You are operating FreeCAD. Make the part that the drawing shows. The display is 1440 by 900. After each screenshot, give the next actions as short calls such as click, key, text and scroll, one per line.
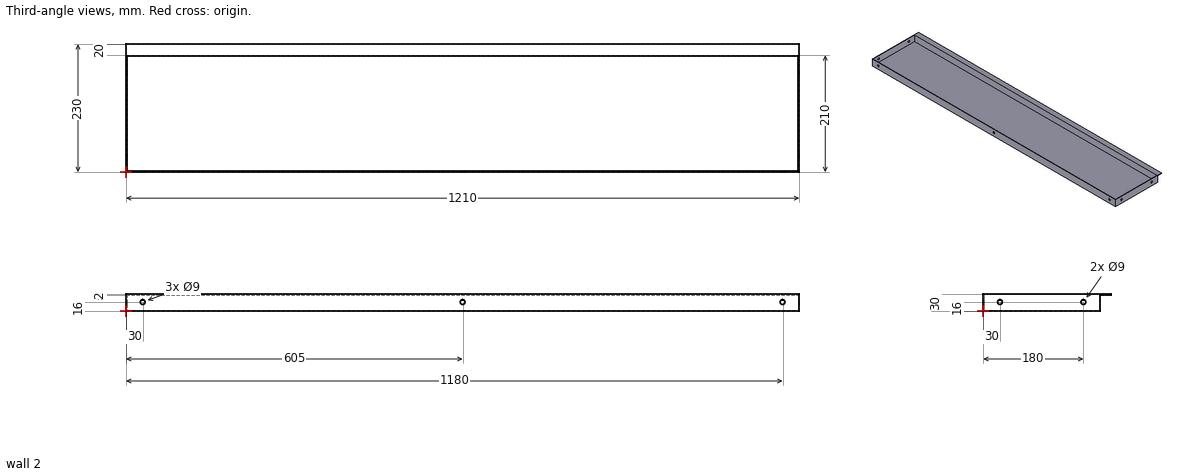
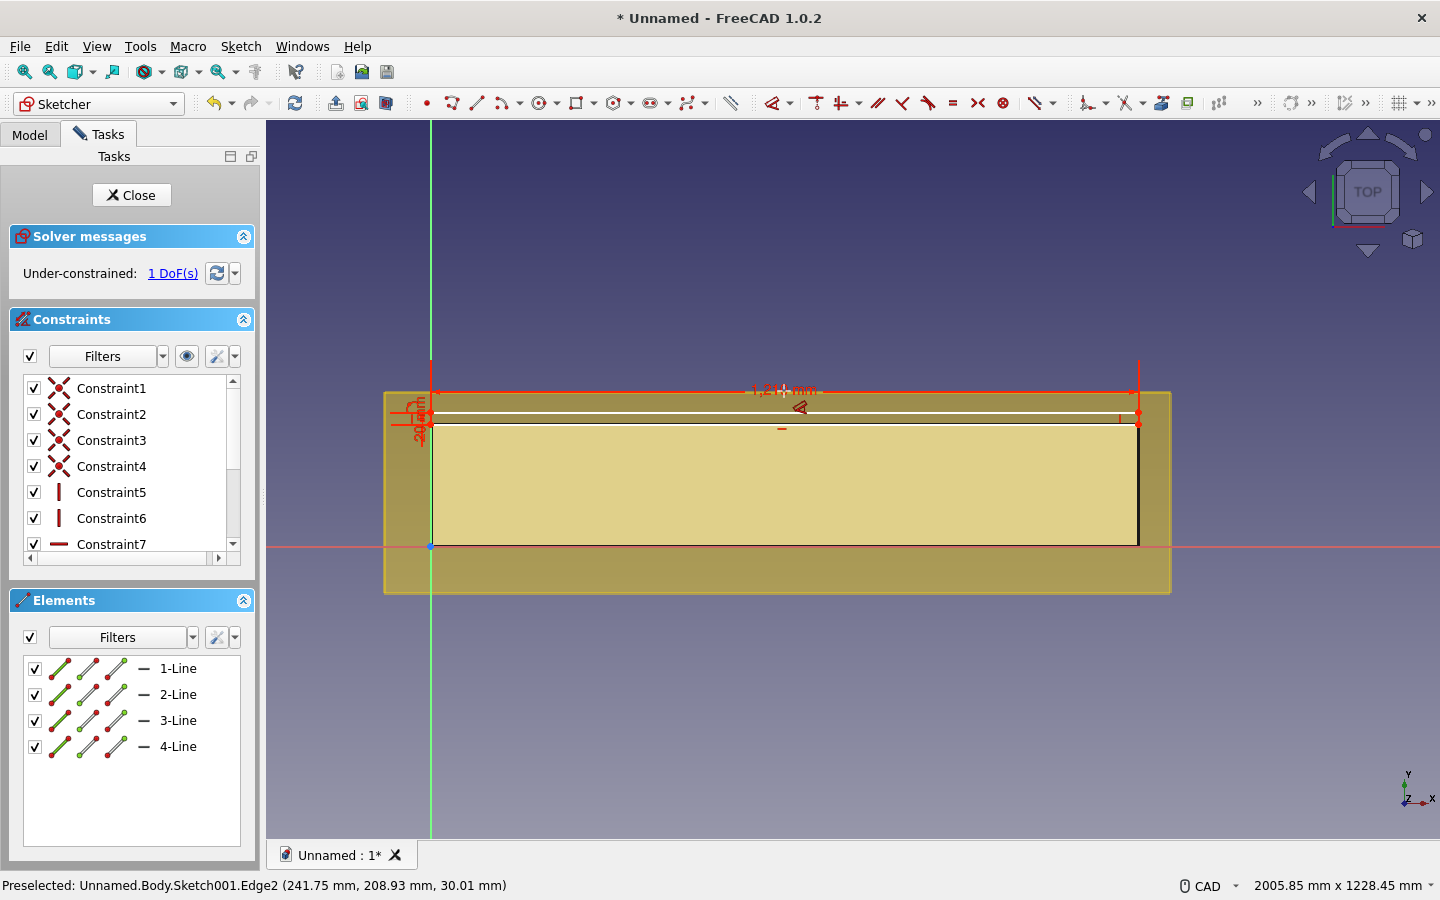
click(431, 413)
click(397, 480)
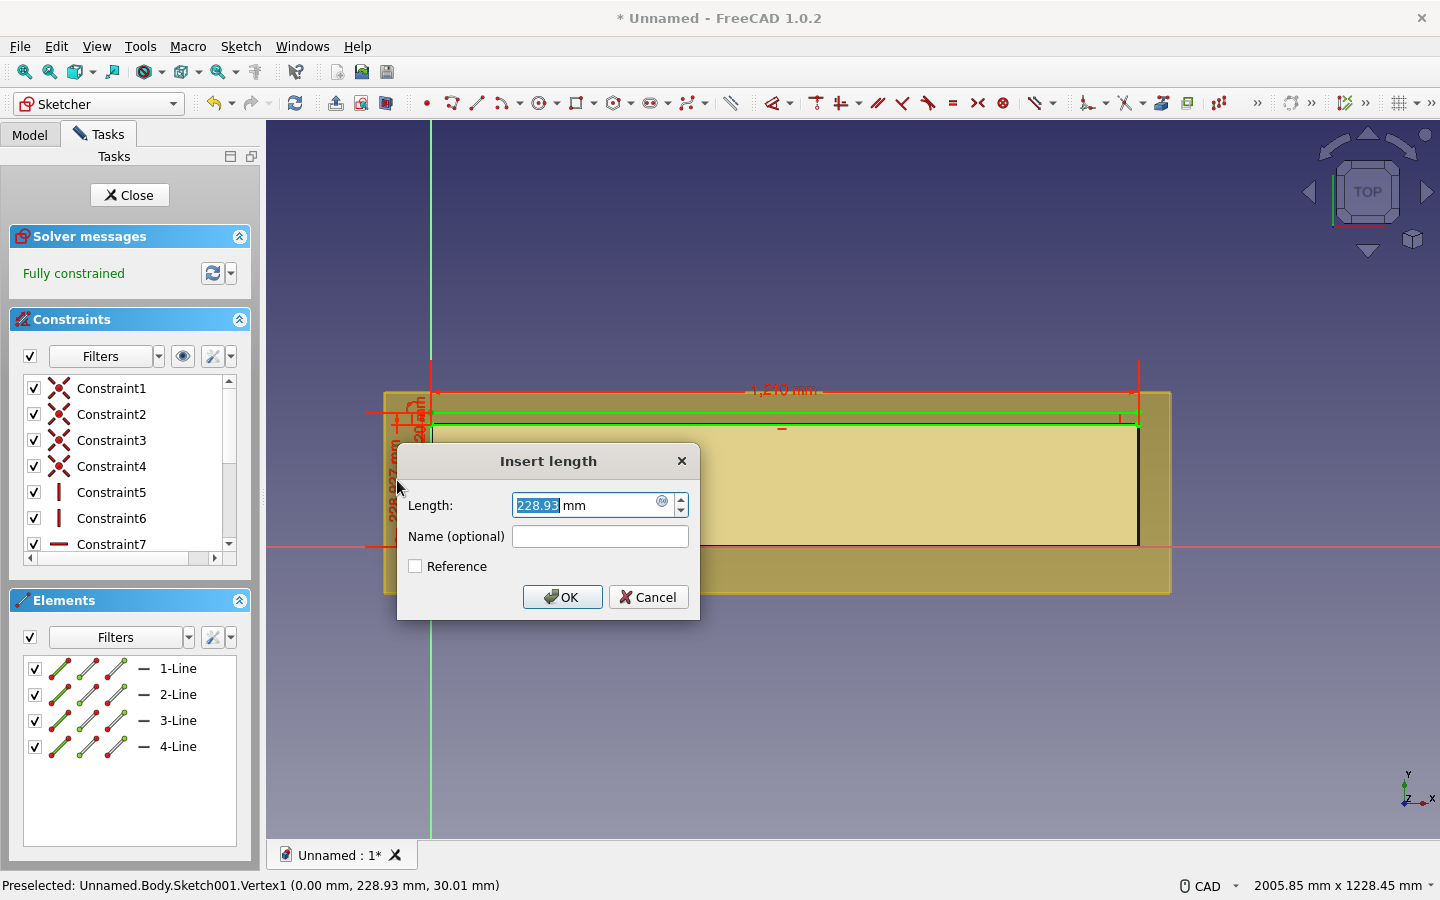
text(230)
key(Return)
key(Escape)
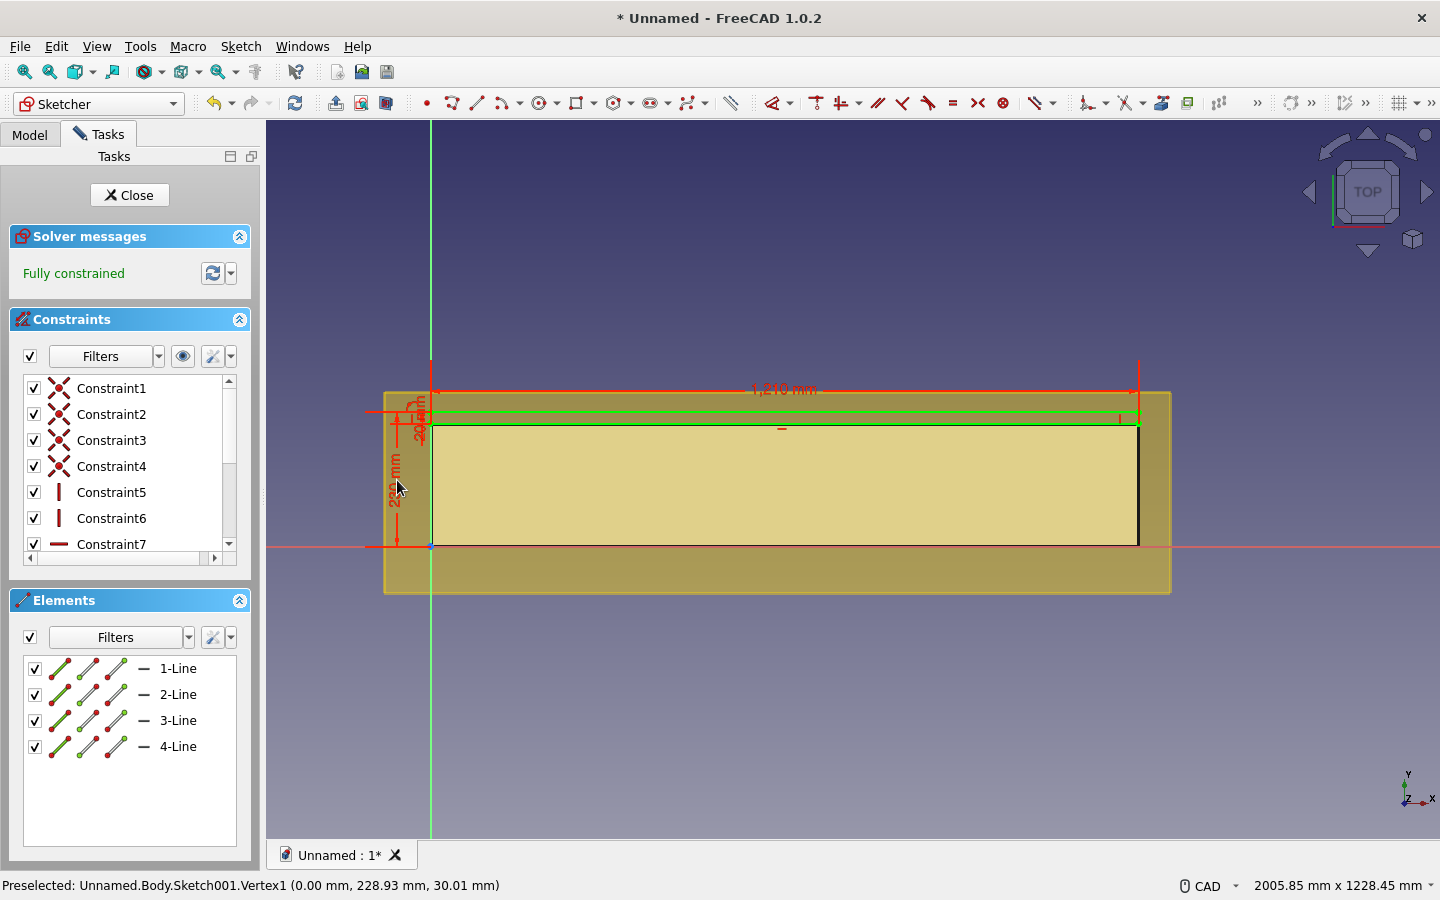
click(130, 195)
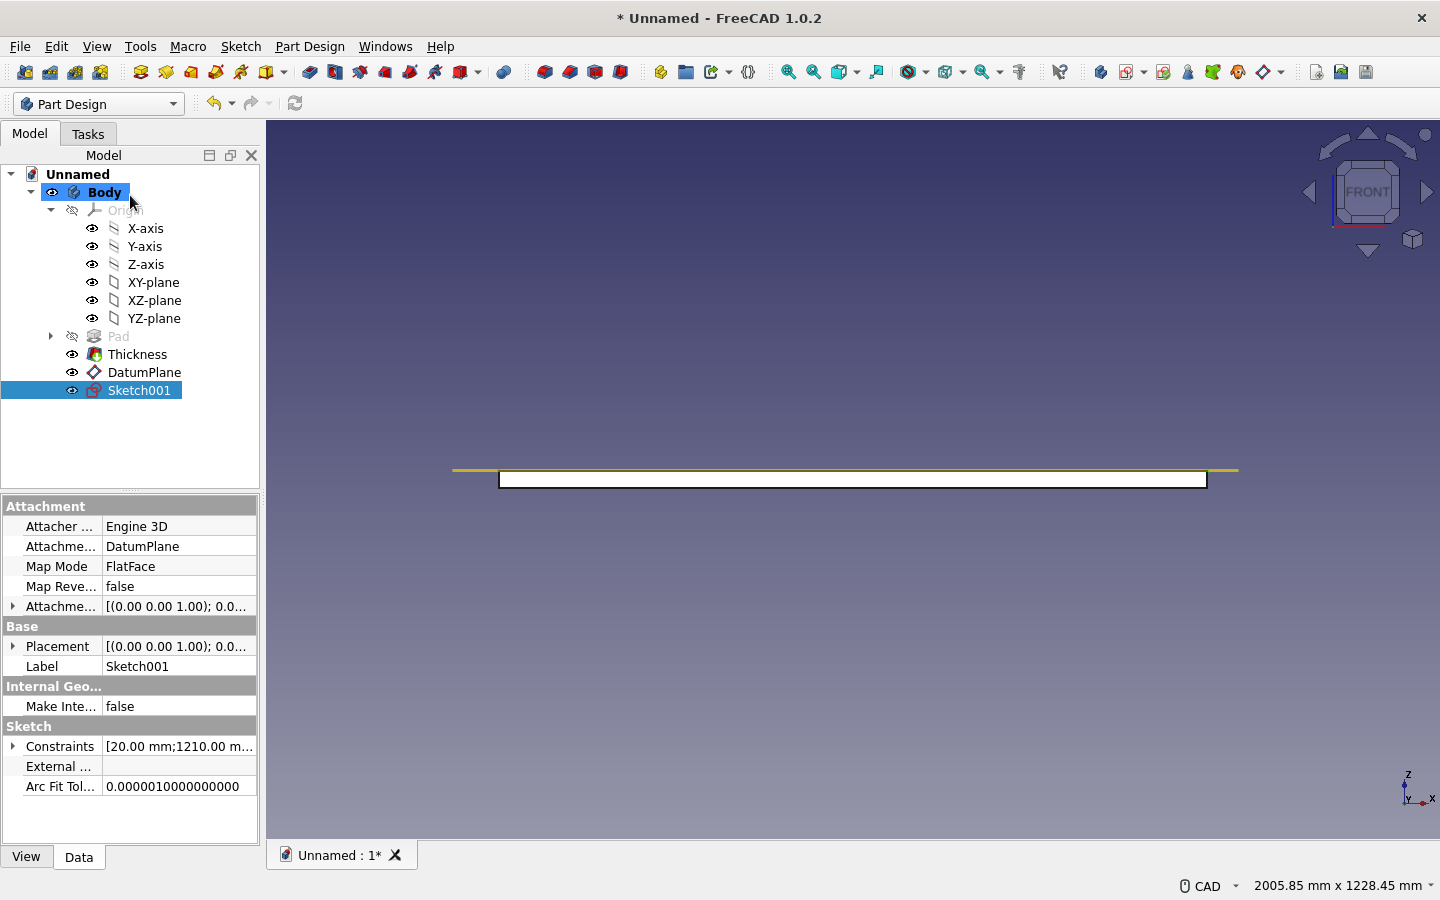
click(141, 72)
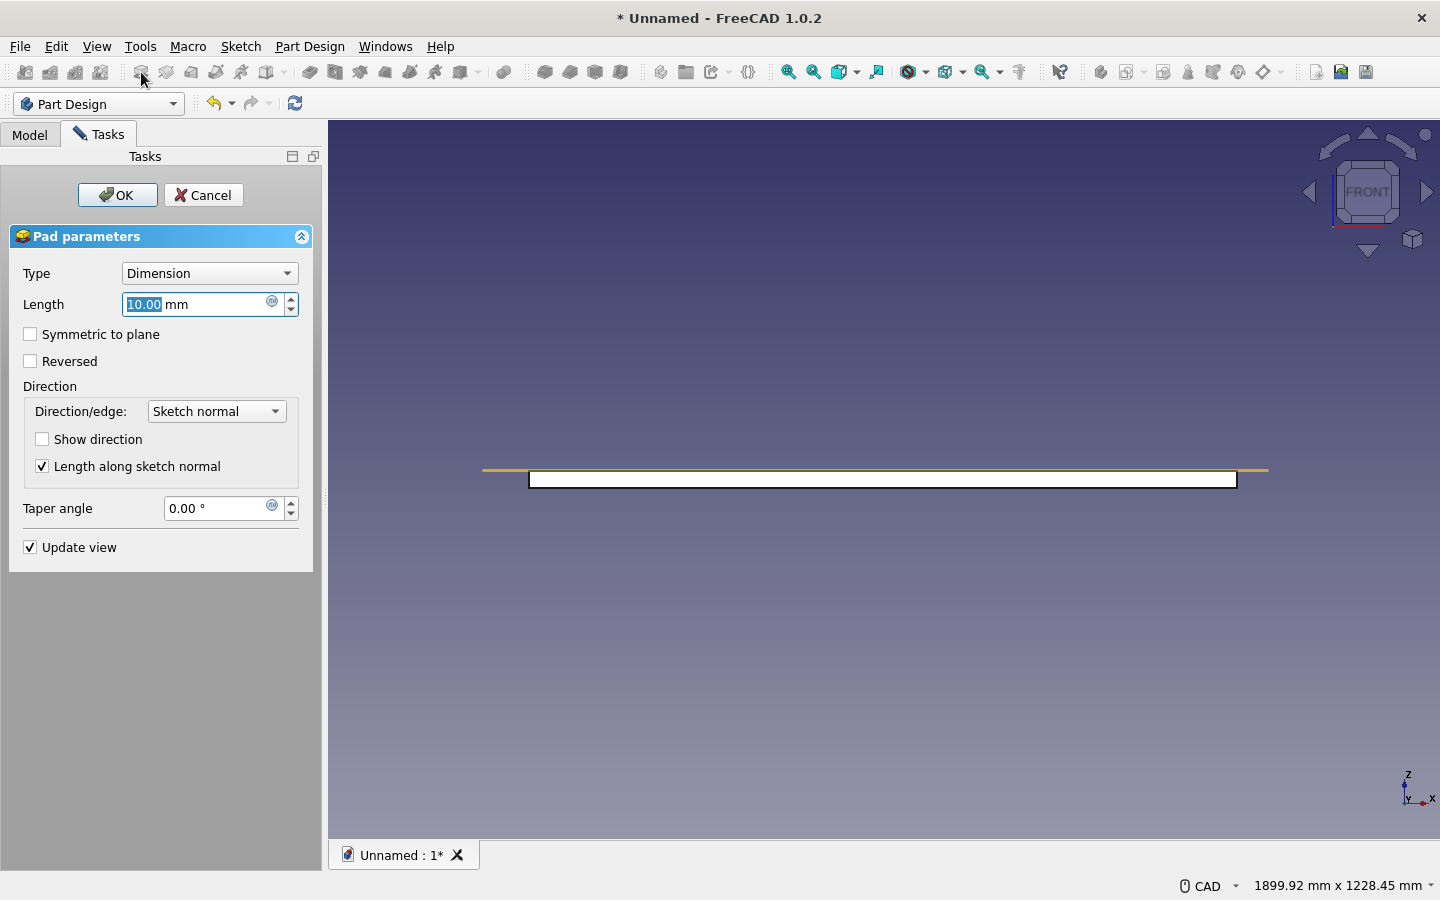
text(2)
key(Tab)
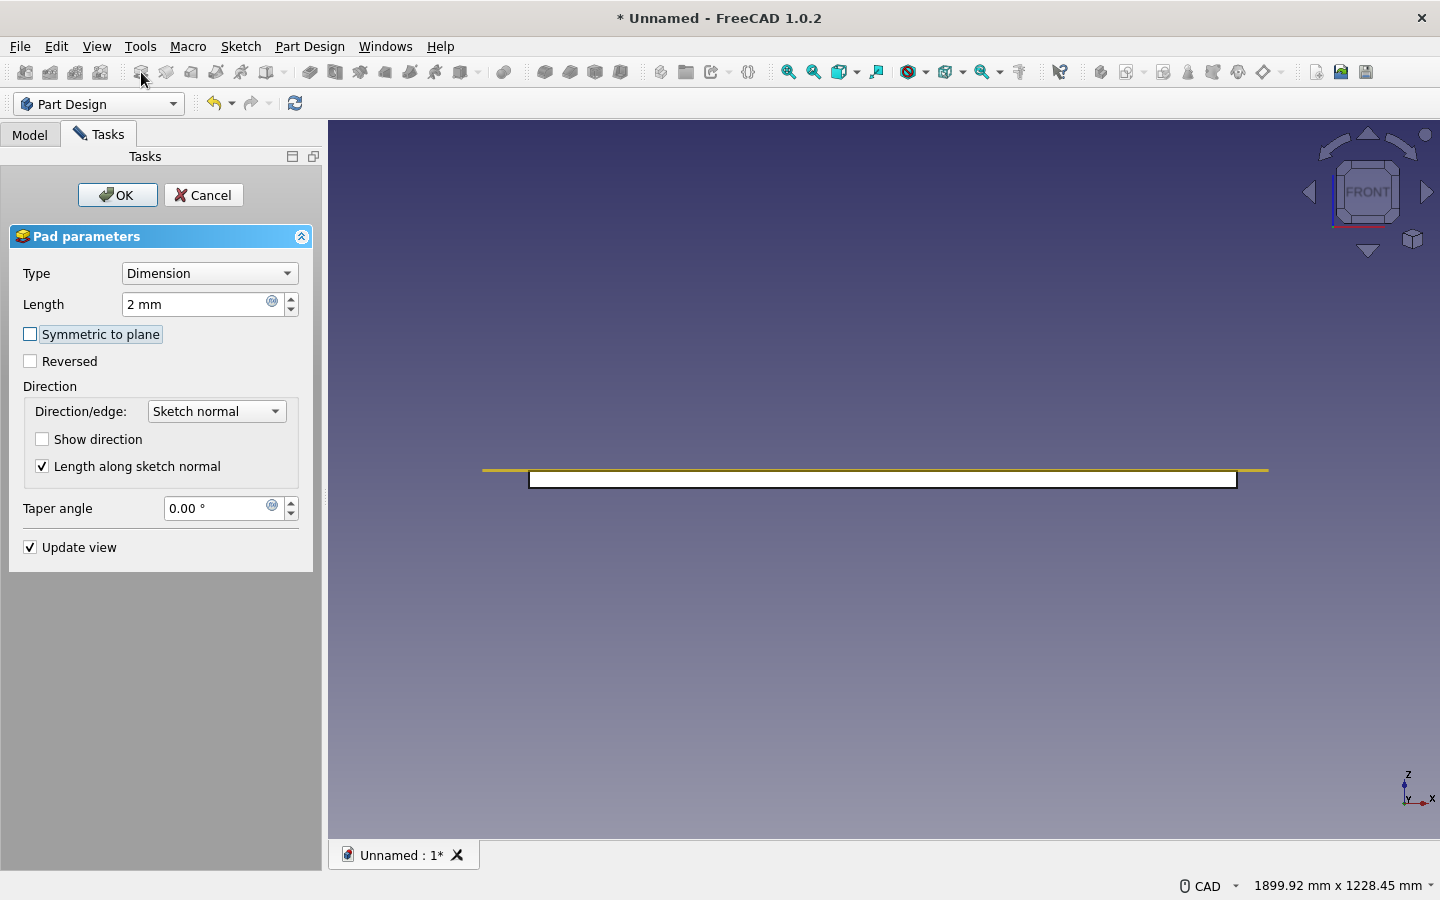
click(31, 361)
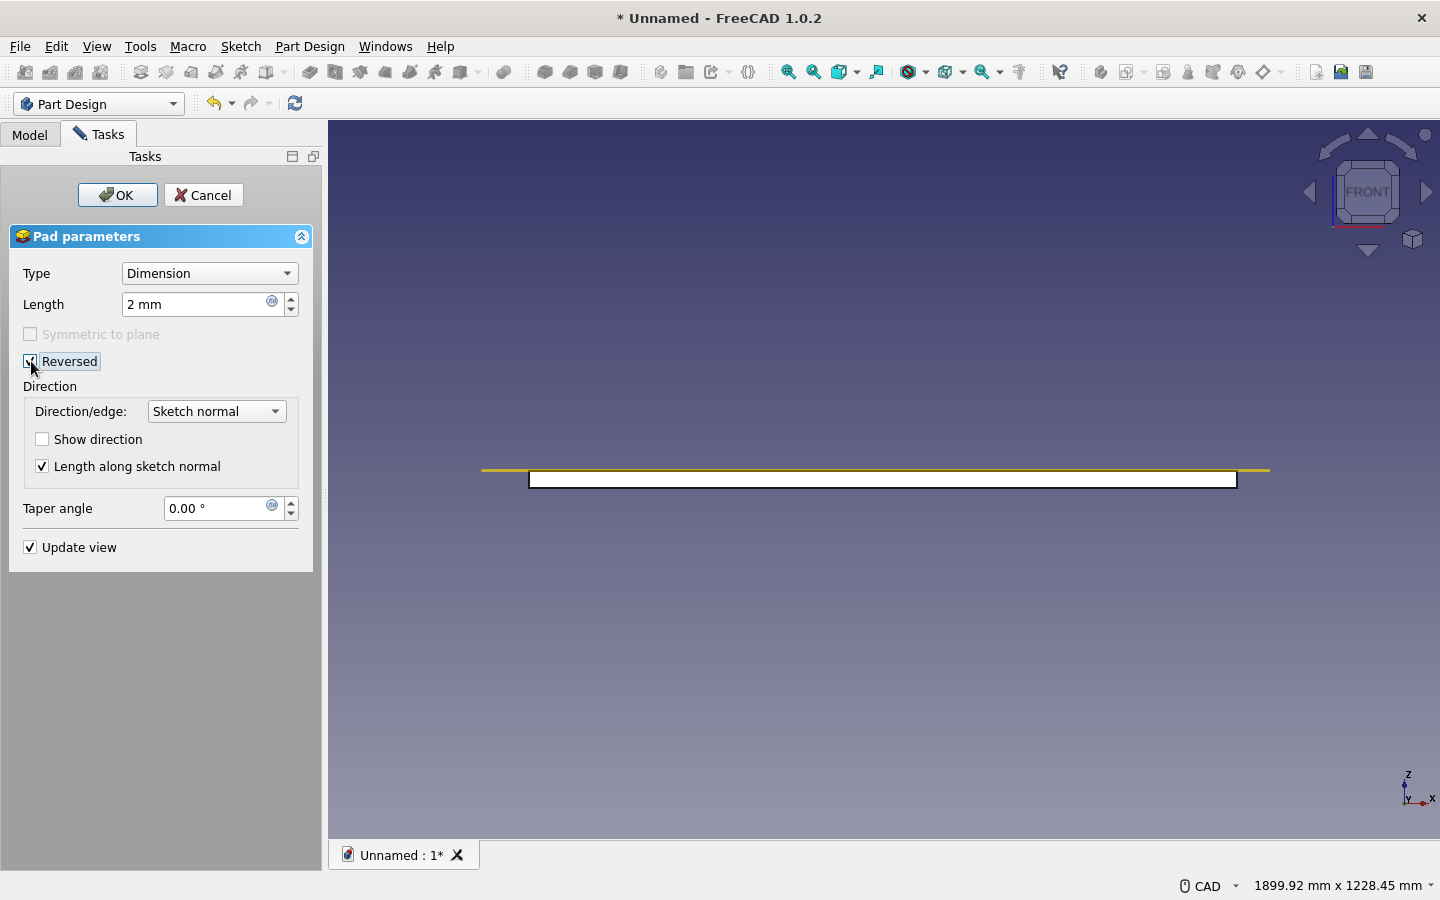
click(118, 195)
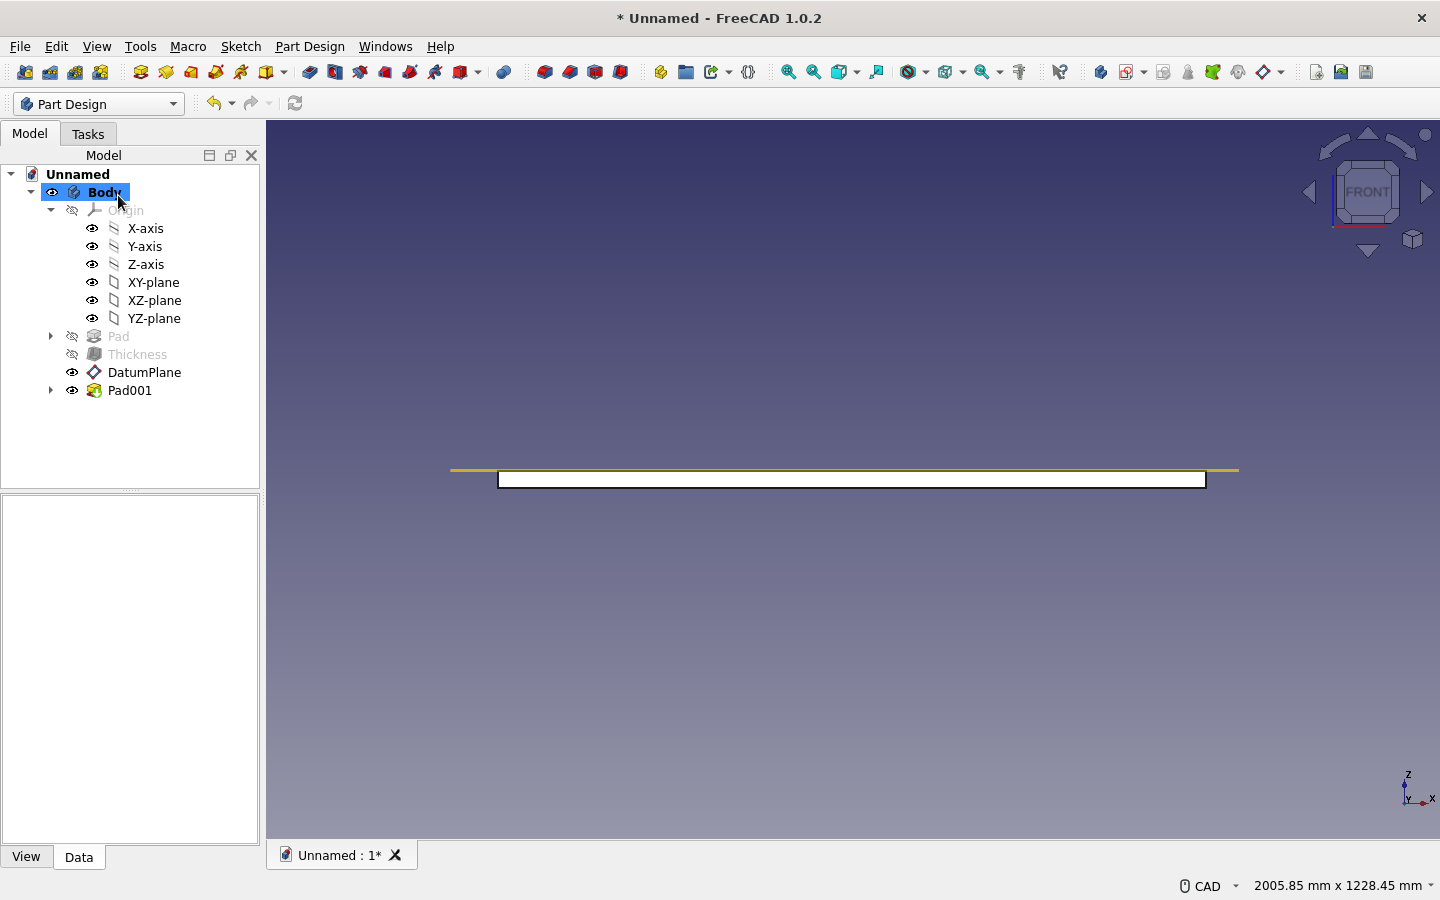
click(117, 372)
key(space)